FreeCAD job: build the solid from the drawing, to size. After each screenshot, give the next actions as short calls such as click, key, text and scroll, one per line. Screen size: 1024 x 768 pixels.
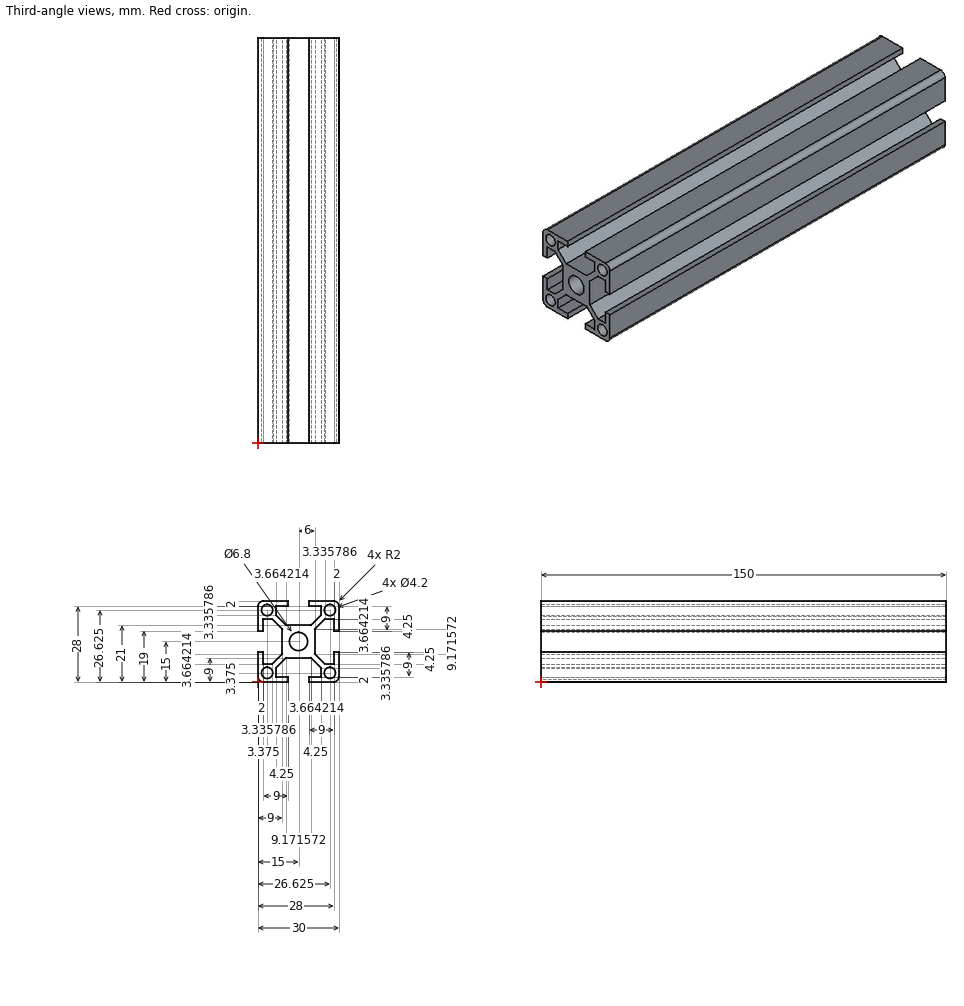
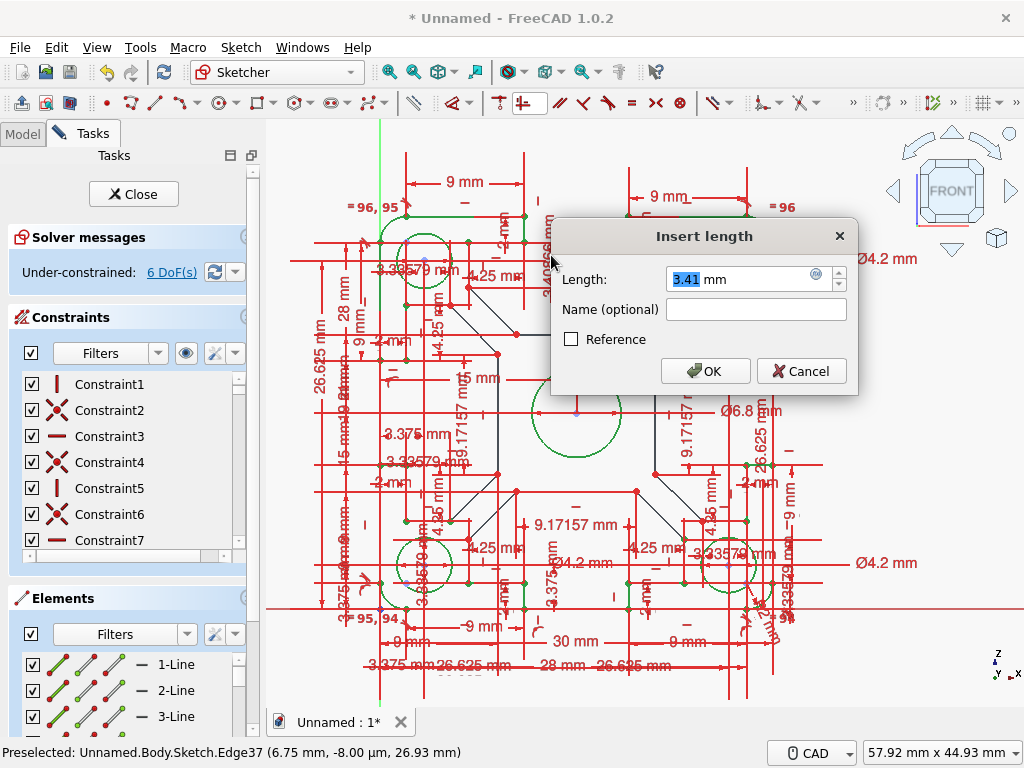
text(3.335786)
key(Return)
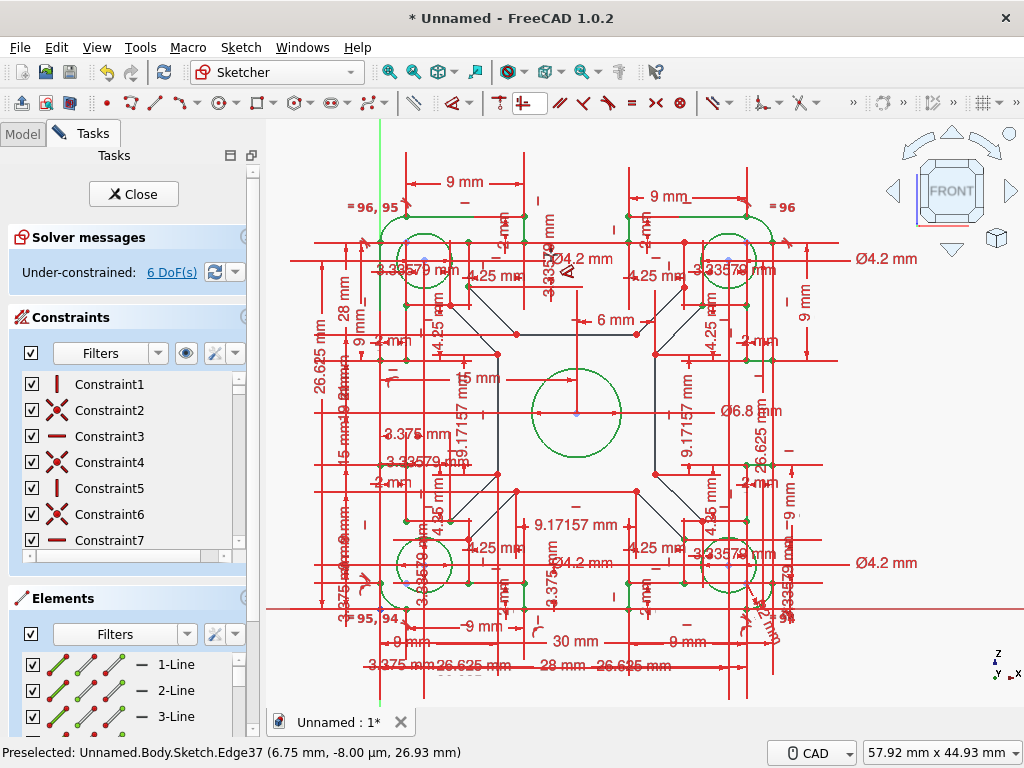
click(552, 335)
click(576, 301)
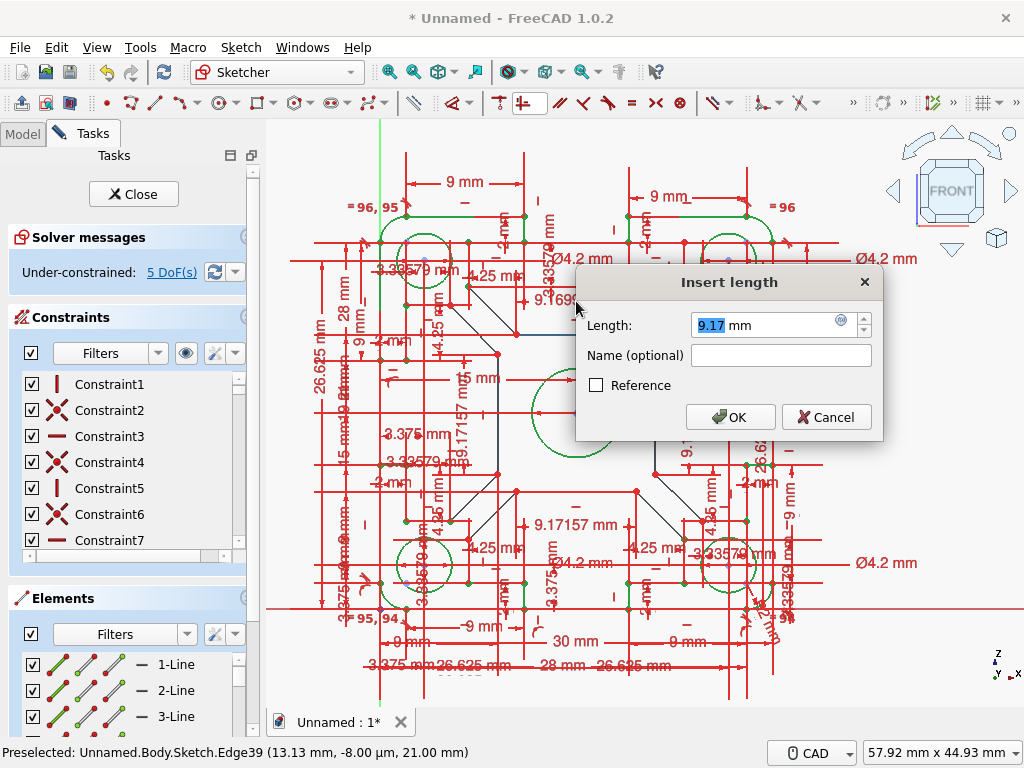
text(9.171572)
key(Return)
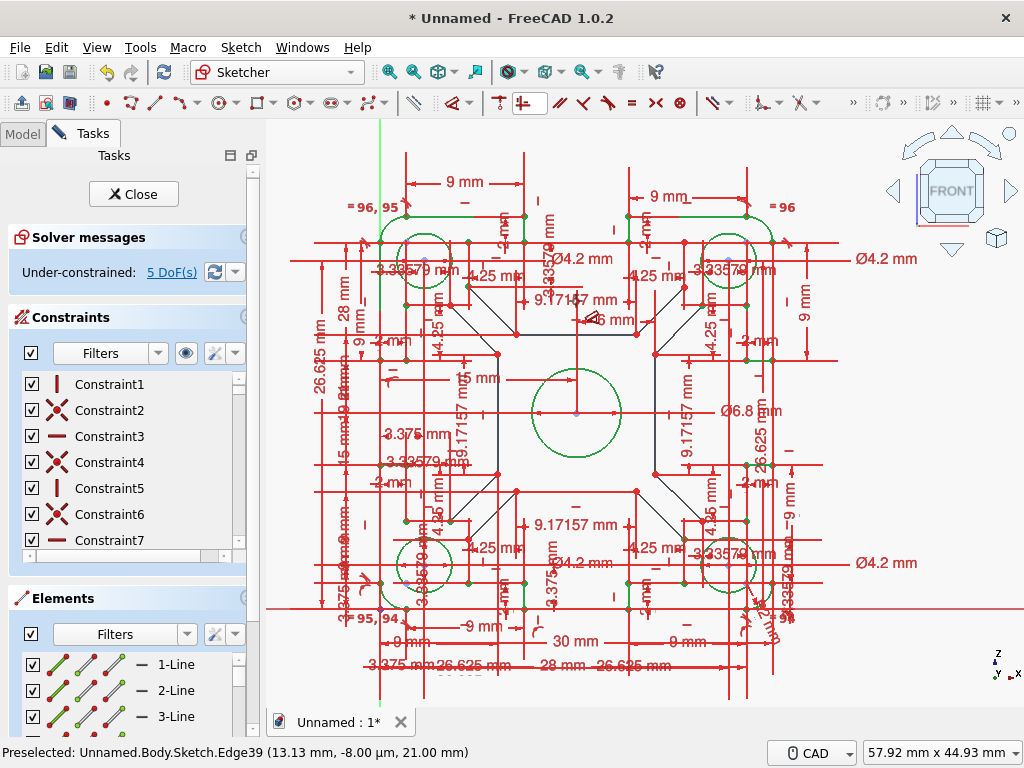
click(684, 274)
click(790, 250)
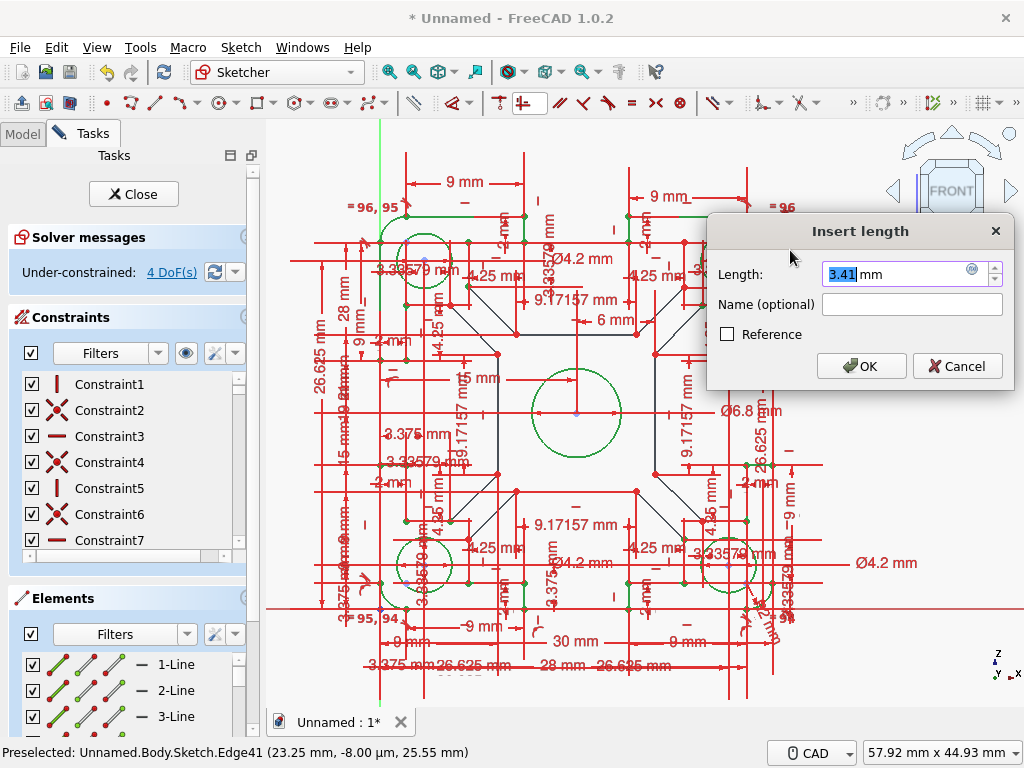
text(3.335786)
key(Return)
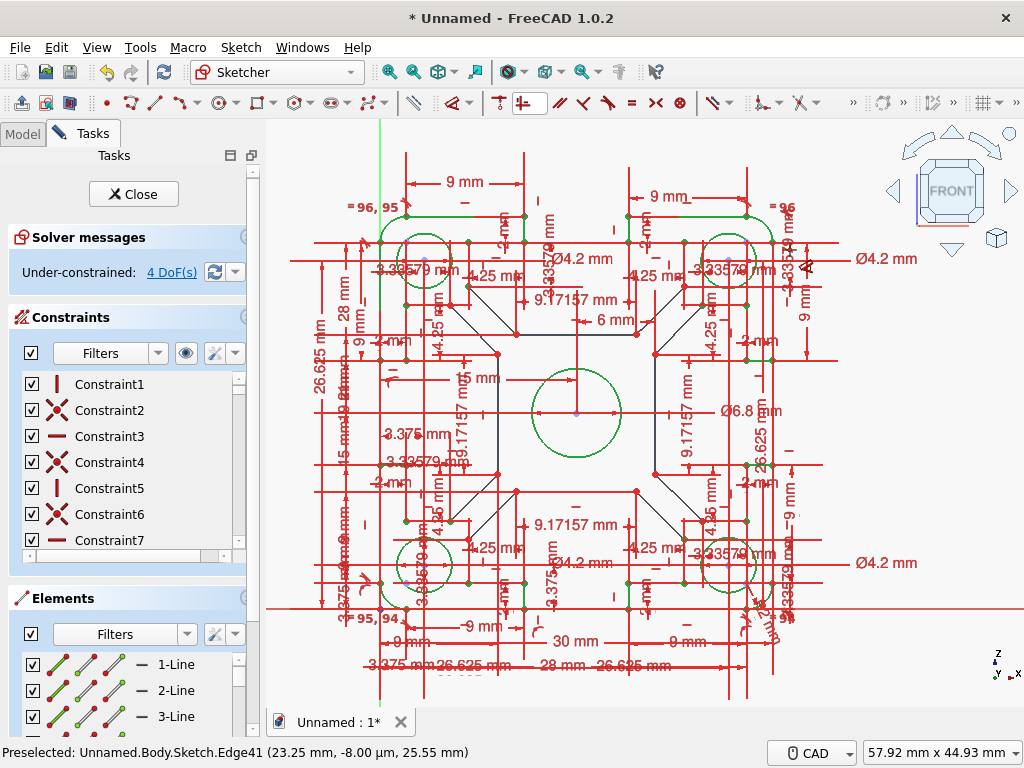
click(689, 320)
click(833, 330)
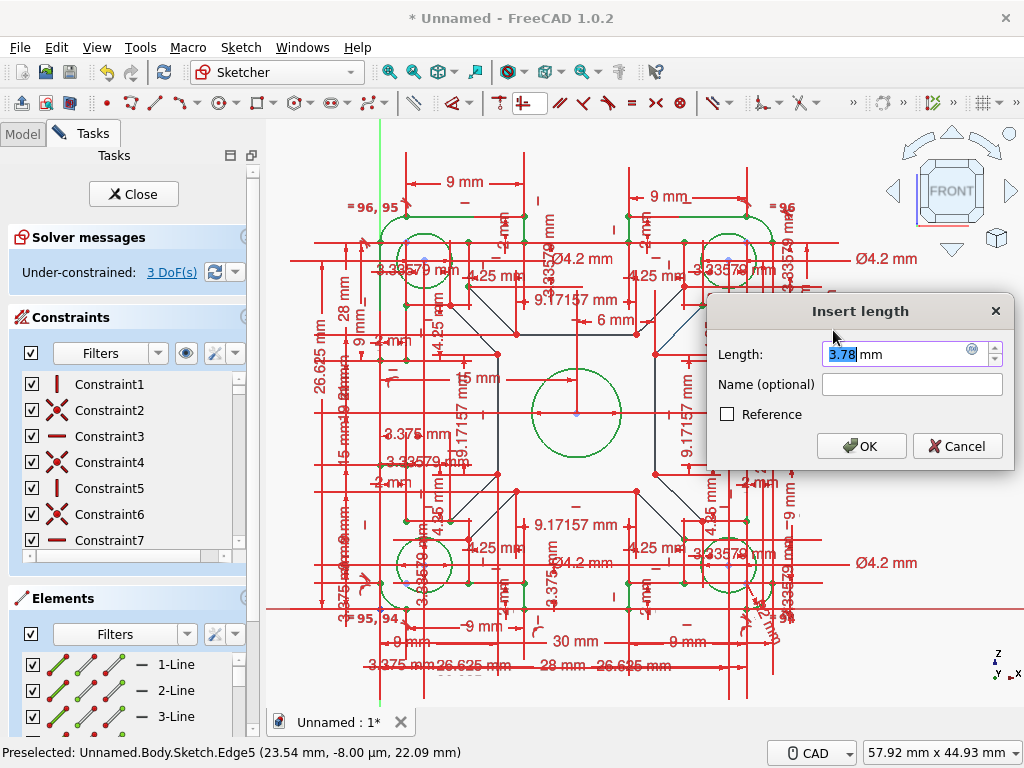
text(3.664214)
key(Return)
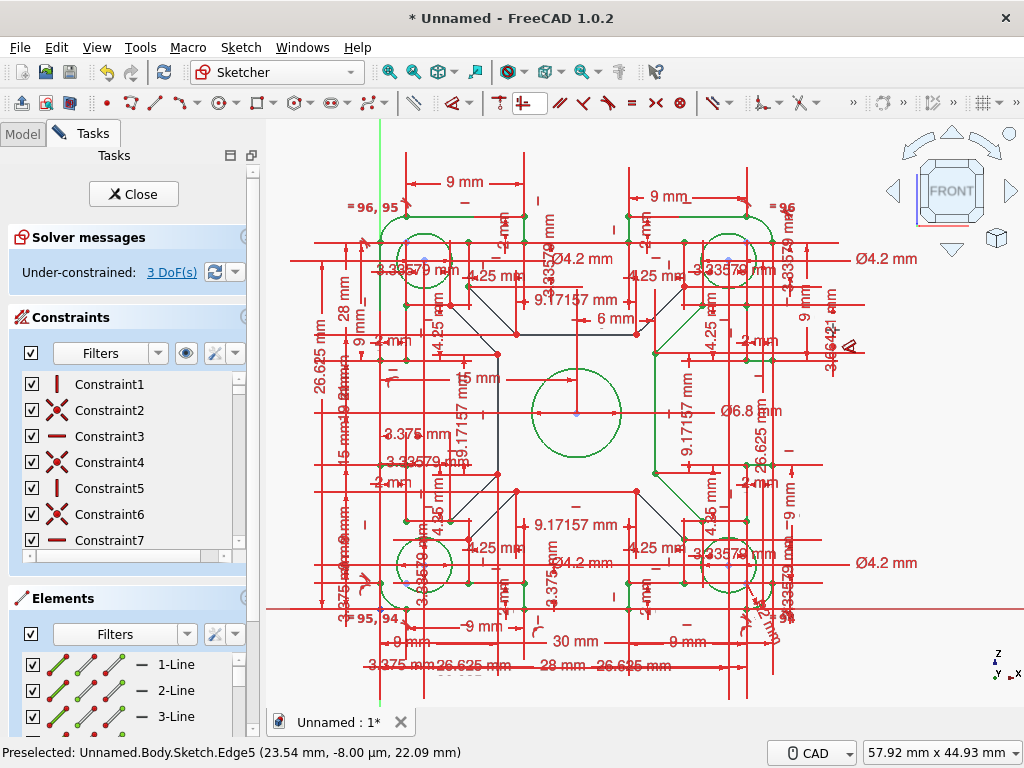
click(670, 525)
click(672, 458)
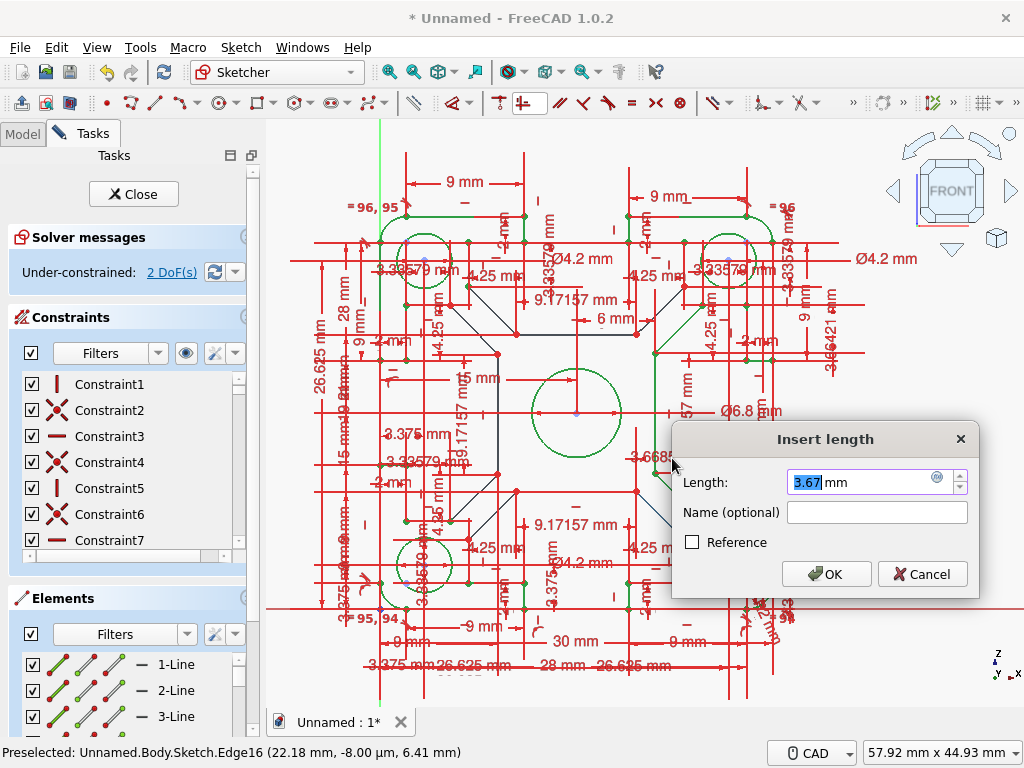
text(3.664214)
key(Return)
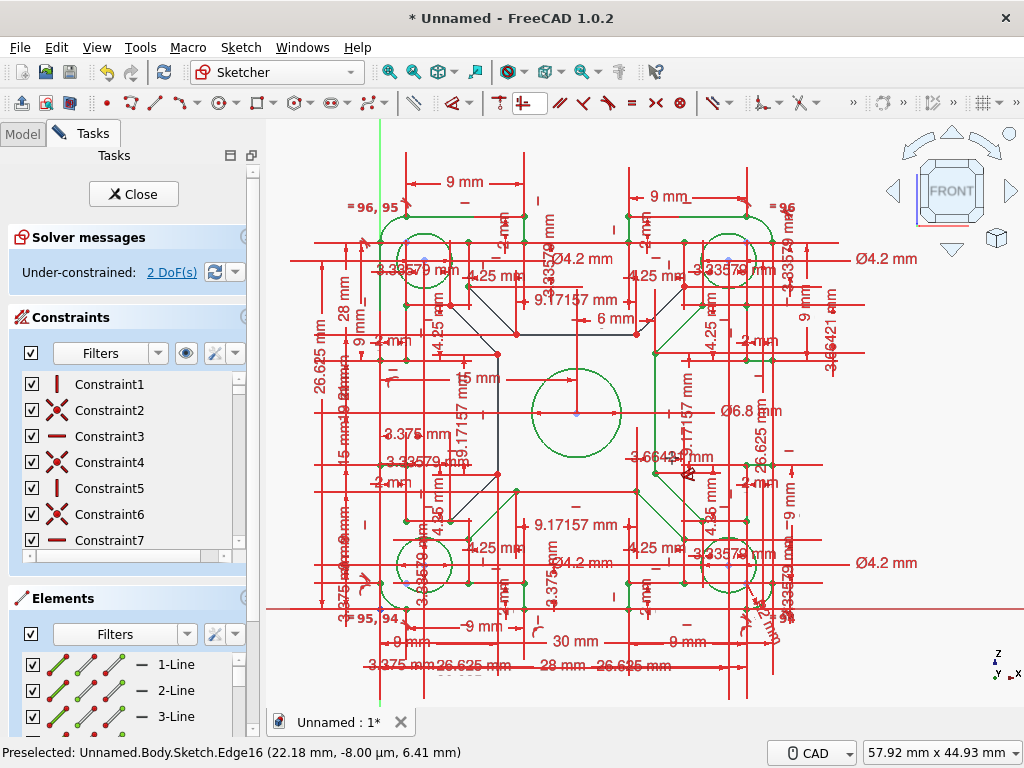
click(464, 507)
click(320, 498)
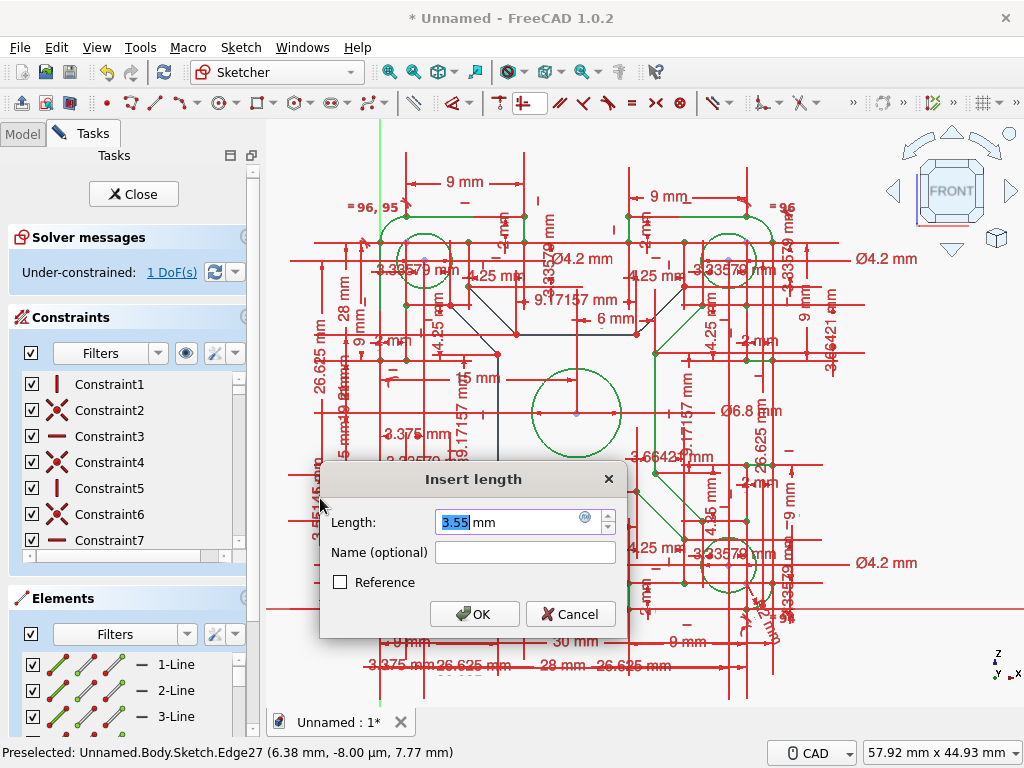
text(3.664214)
key(Return)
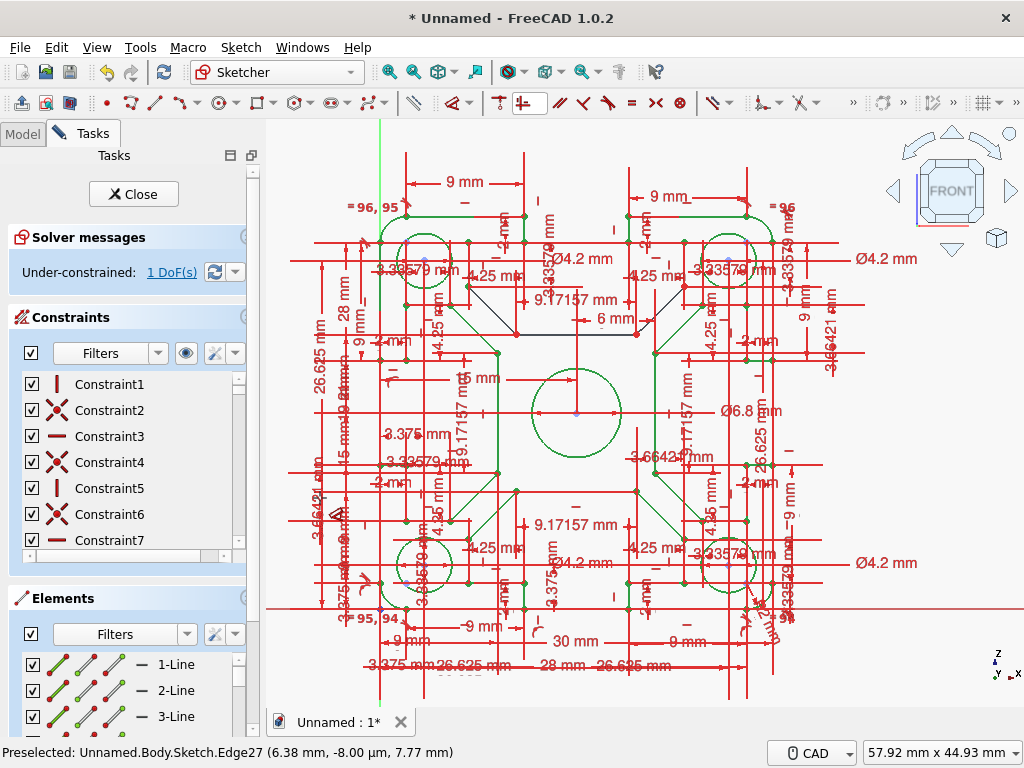
click(483, 301)
click(492, 157)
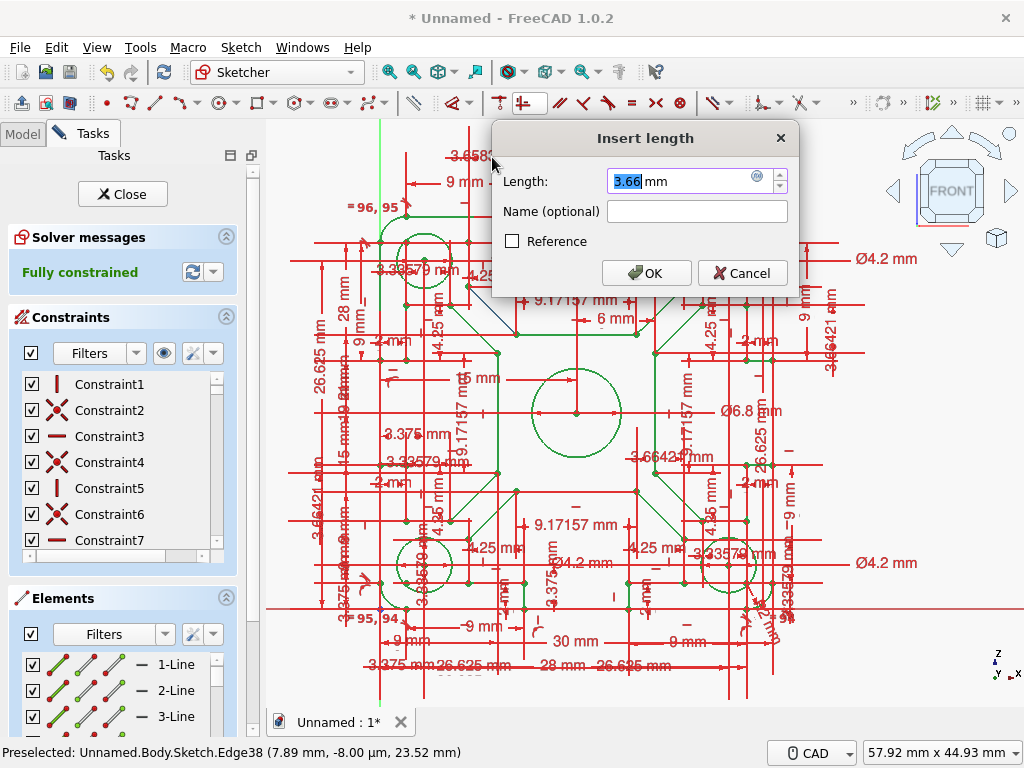
text(3.664214)
key(Return)
key(Escape)